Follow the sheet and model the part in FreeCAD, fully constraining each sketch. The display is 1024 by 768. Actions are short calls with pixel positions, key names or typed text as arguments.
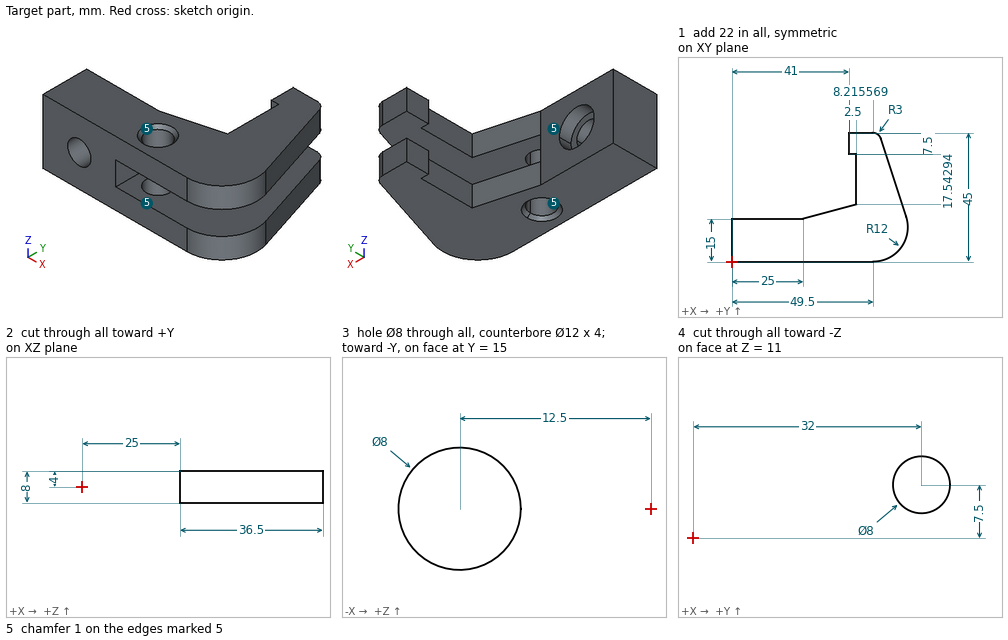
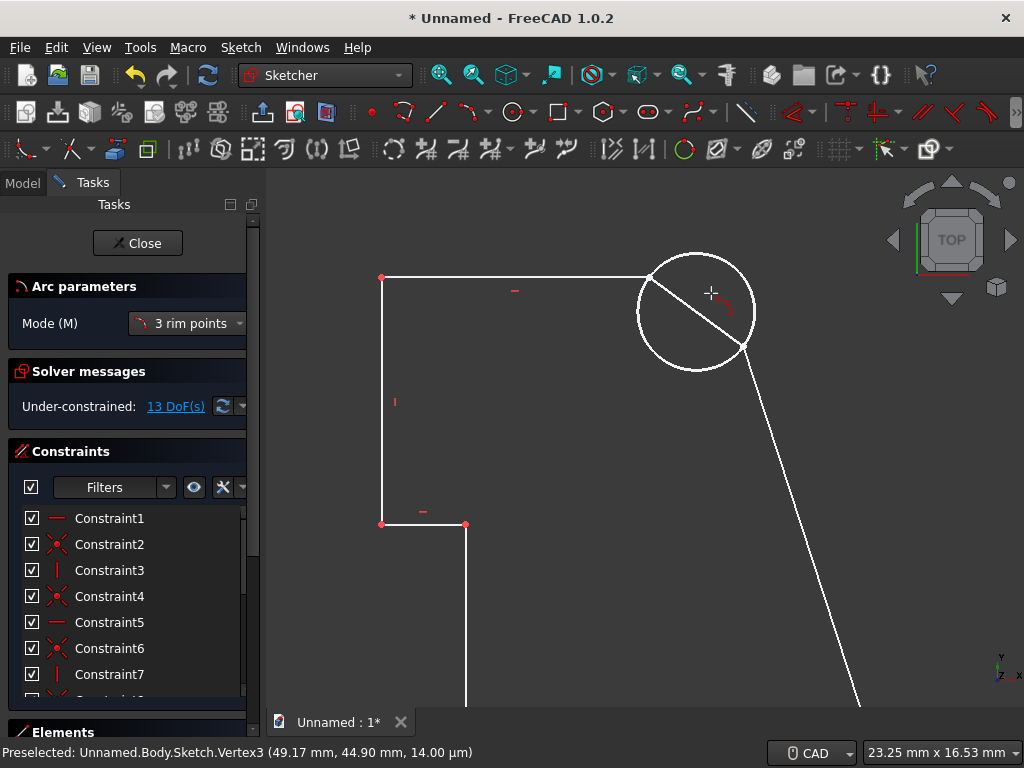
click(708, 293)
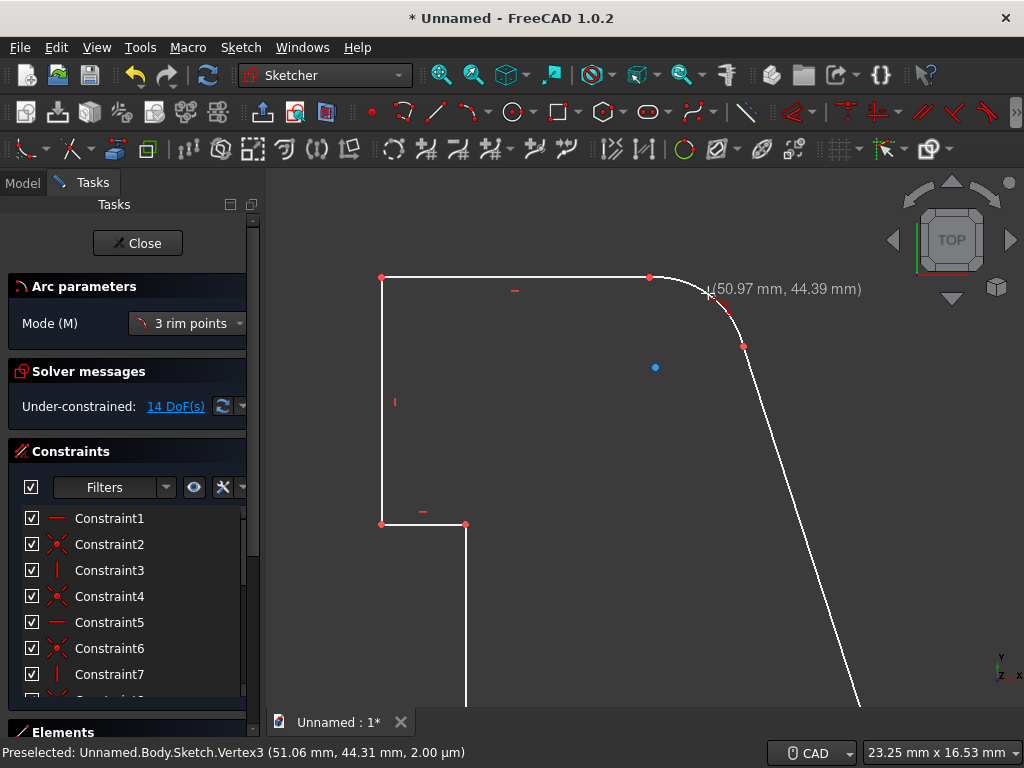
scroll(712, 293, down, 8)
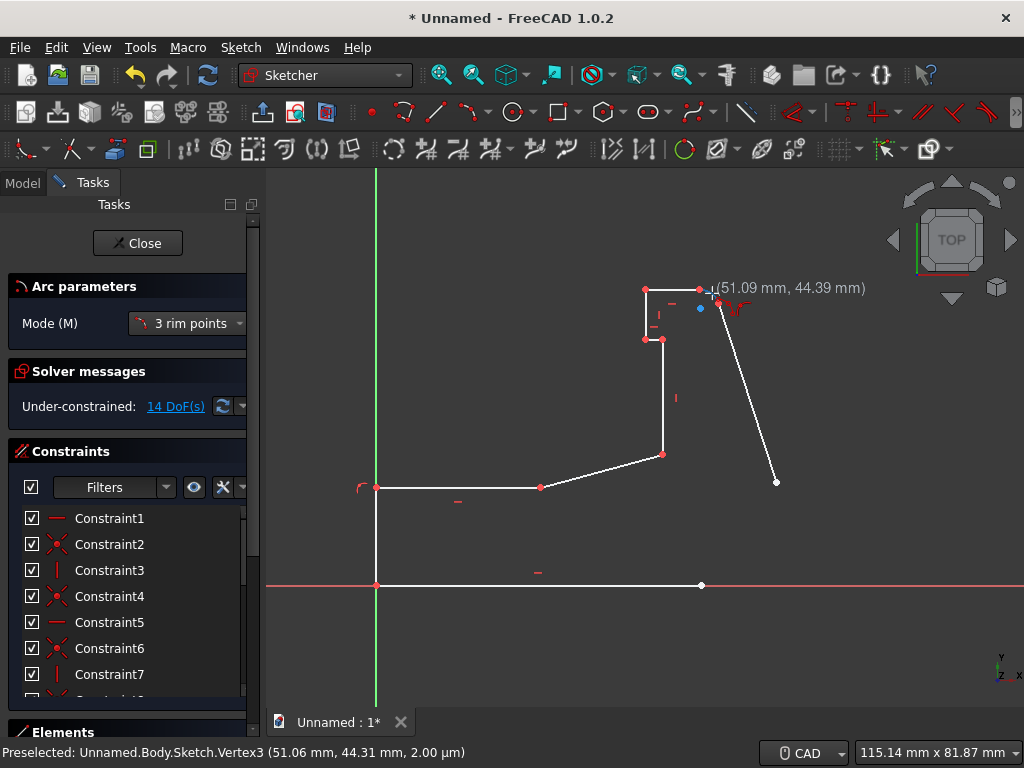
click(702, 586)
click(777, 483)
click(766, 553)
key(Escape)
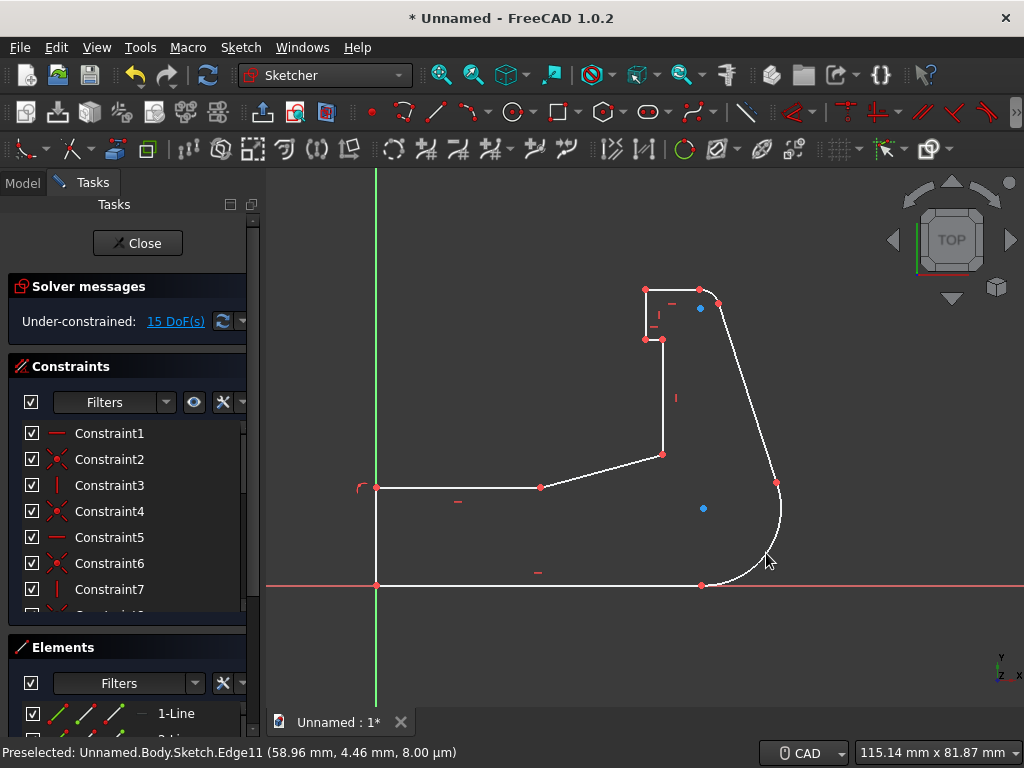
click(759, 429)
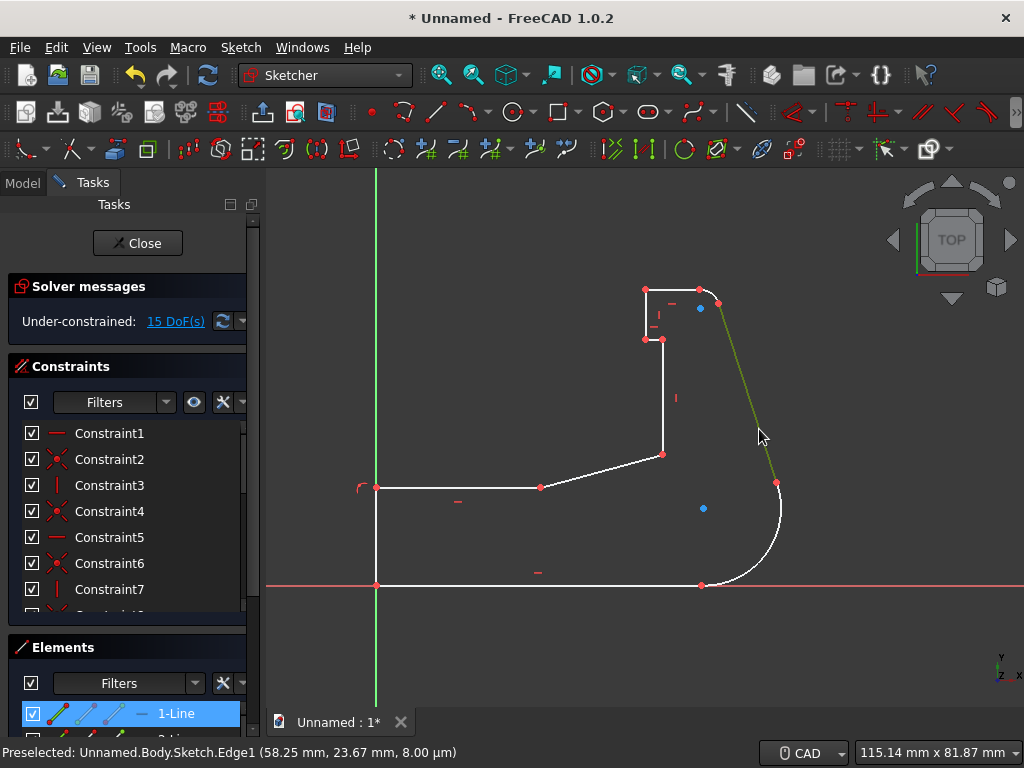
click(712, 294)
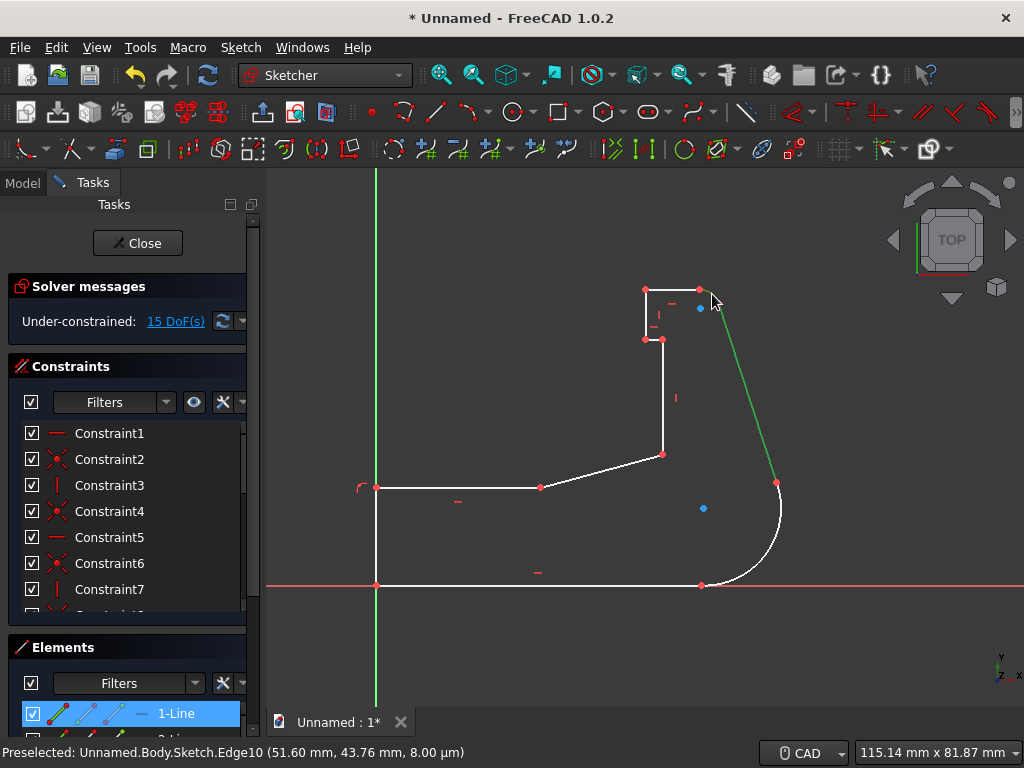
key(t)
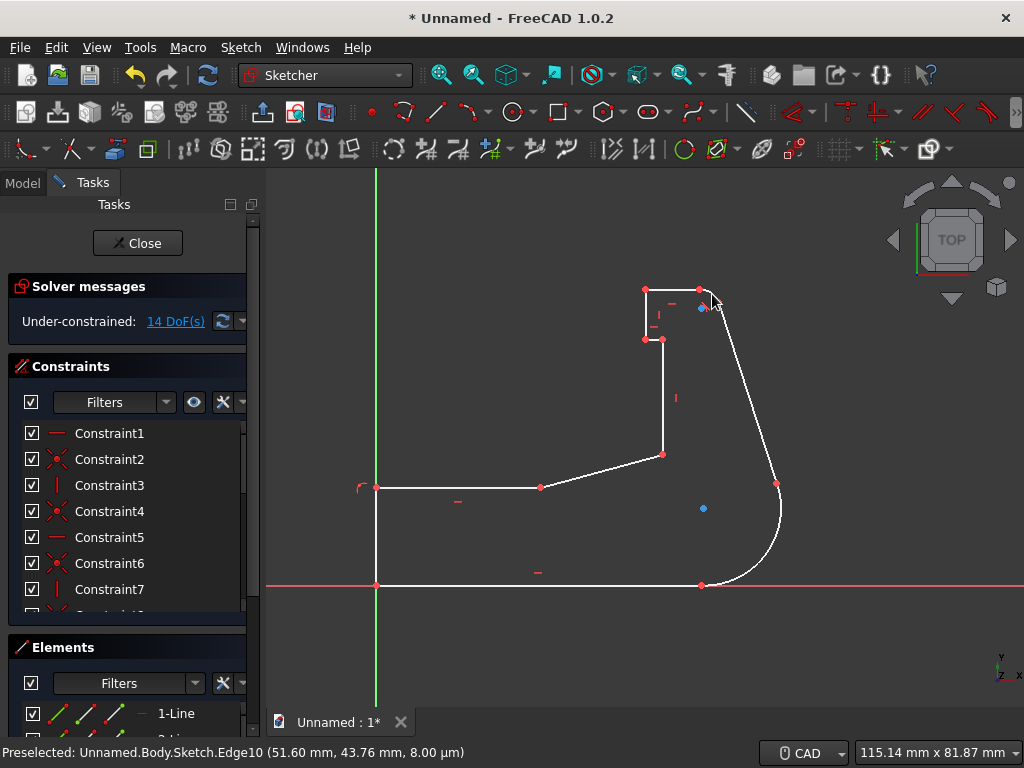
click(759, 429)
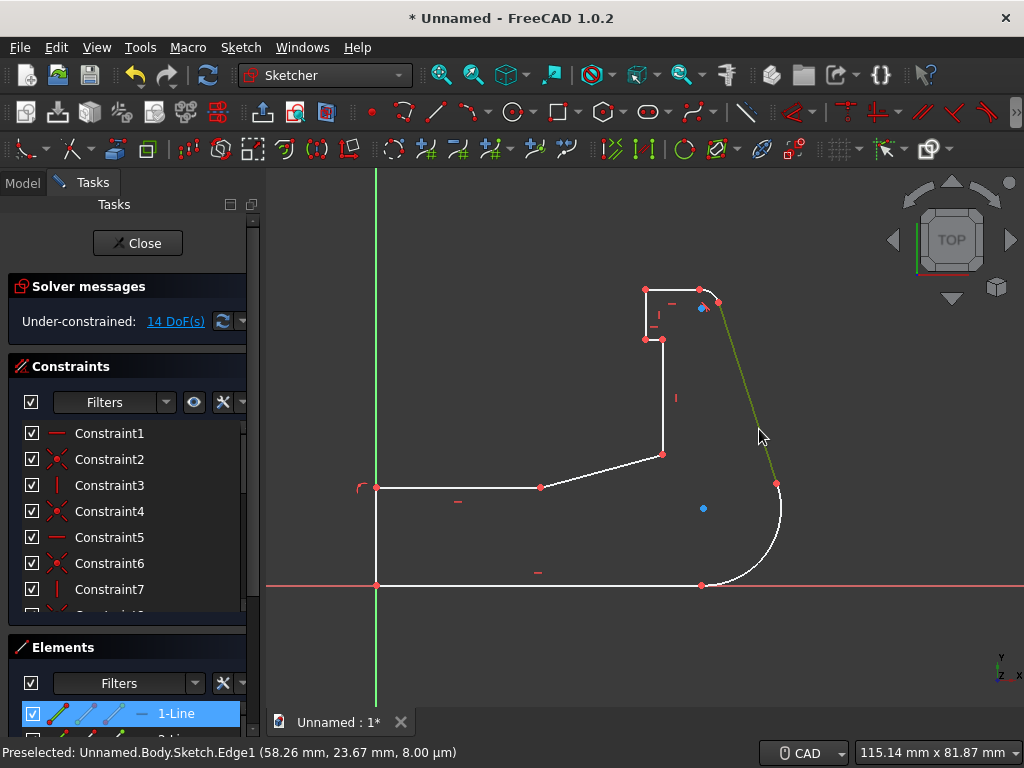
click(744, 574)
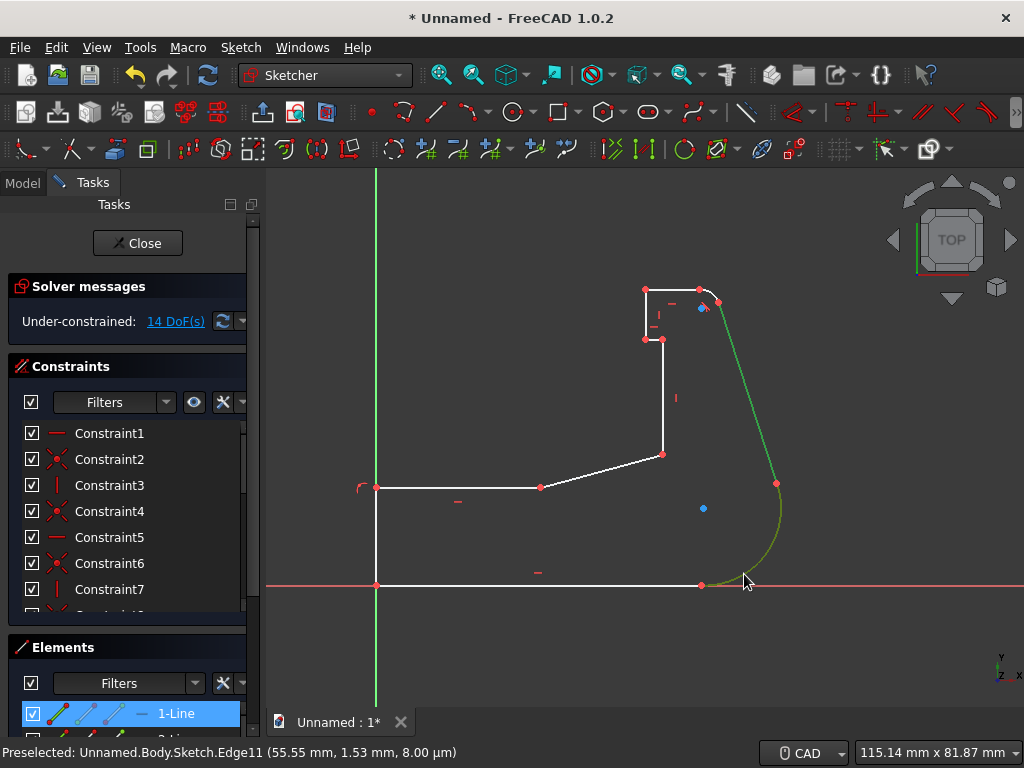
click(988, 112)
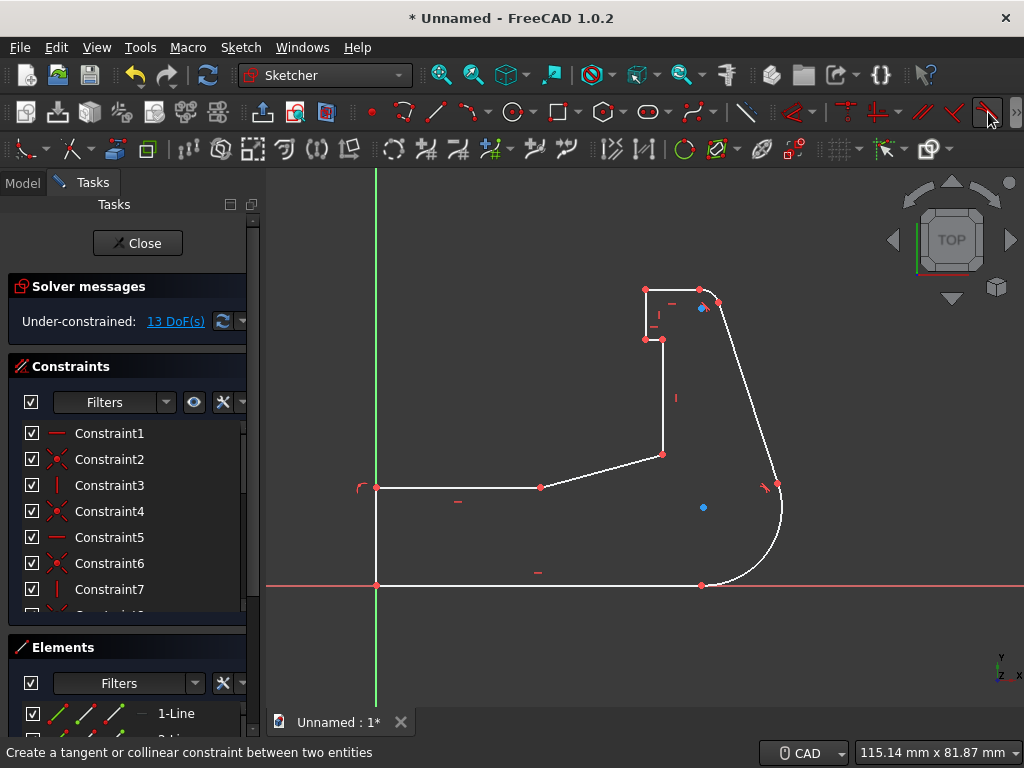
click(684, 290)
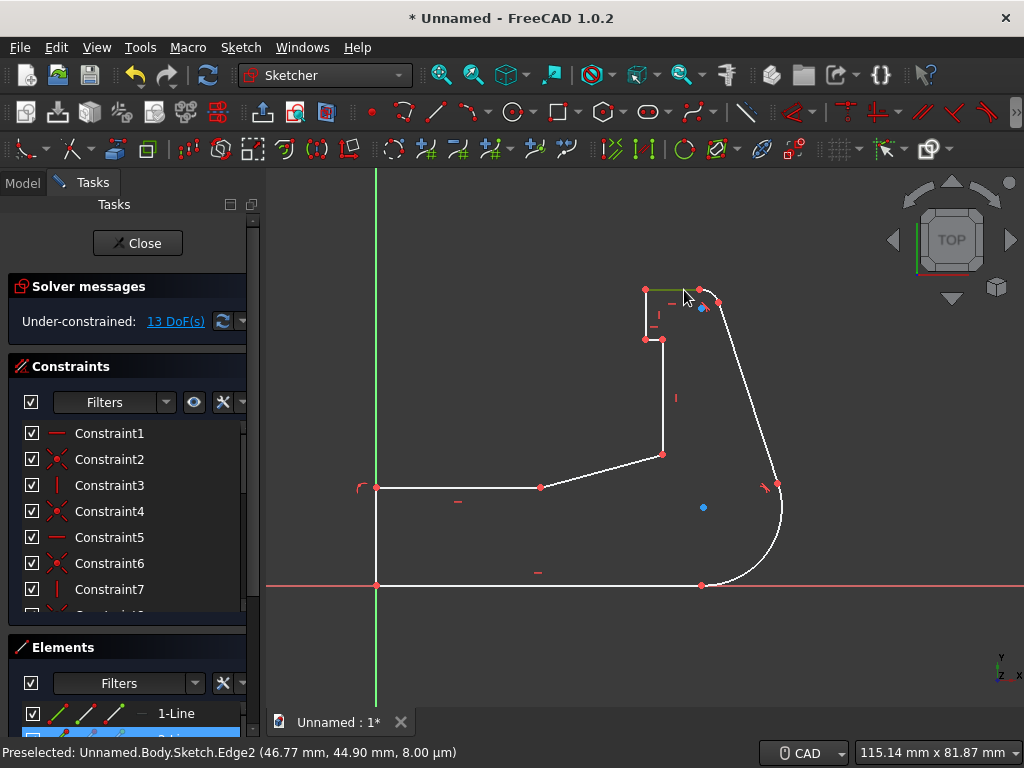
click(711, 293)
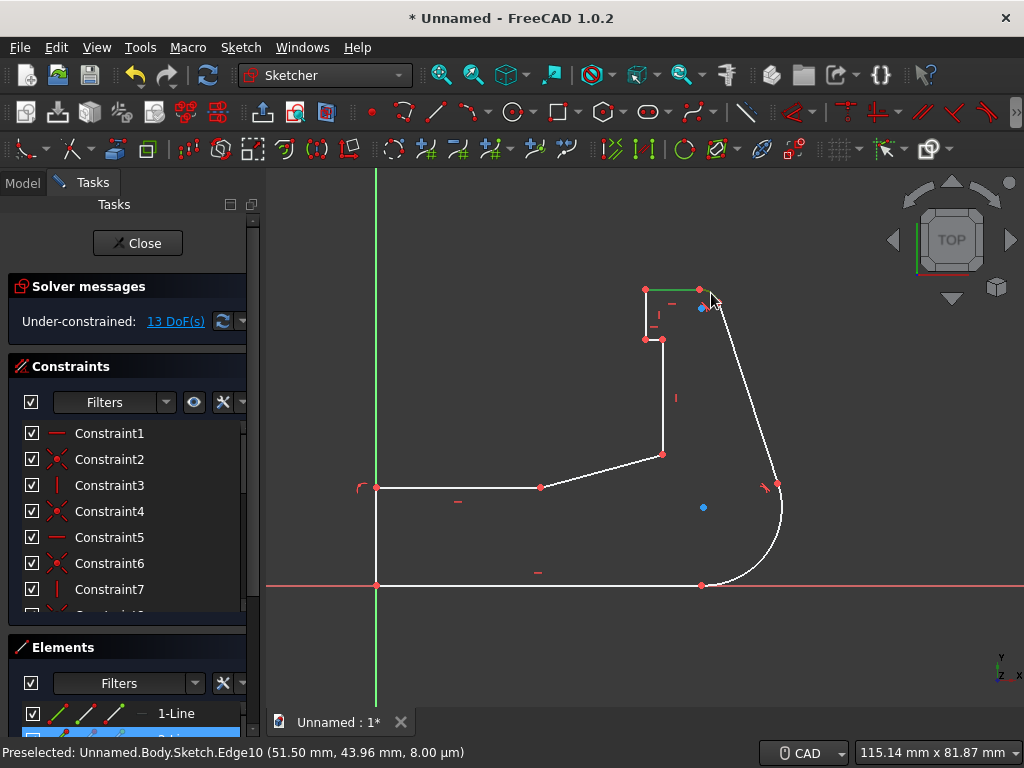
key(t)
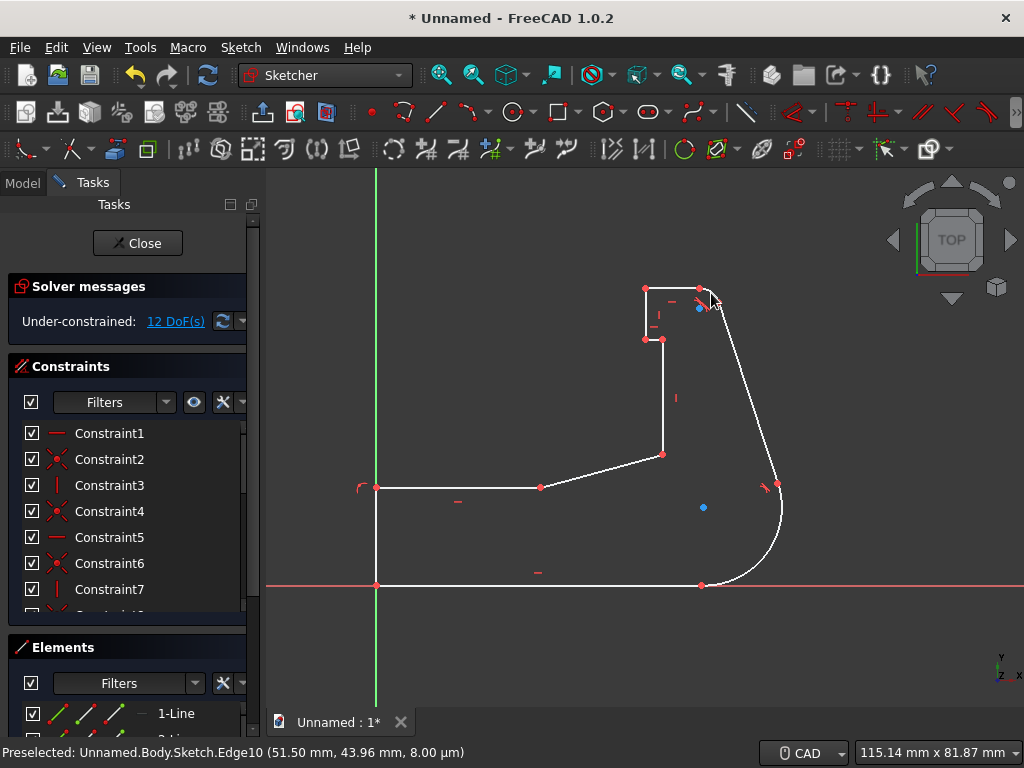
click(474, 586)